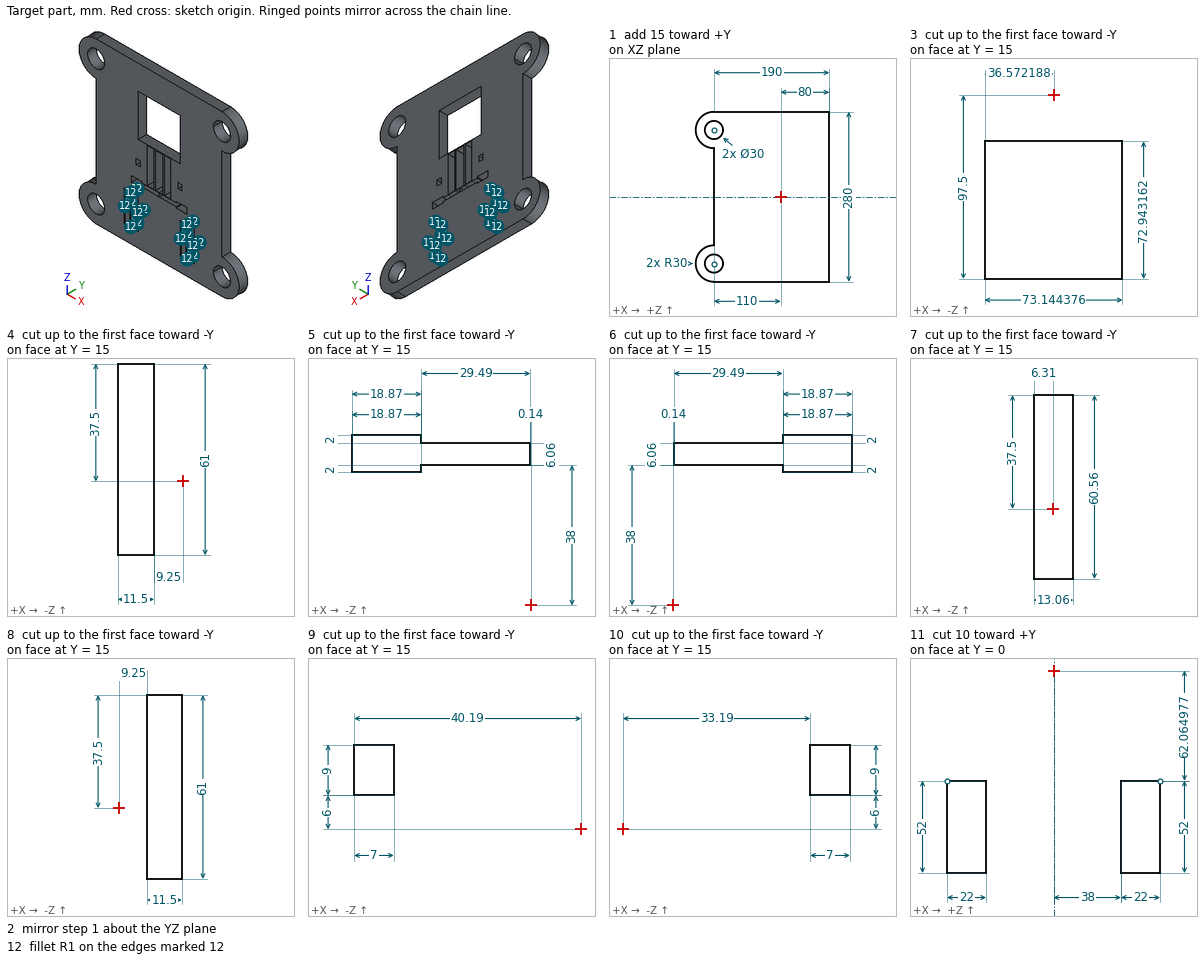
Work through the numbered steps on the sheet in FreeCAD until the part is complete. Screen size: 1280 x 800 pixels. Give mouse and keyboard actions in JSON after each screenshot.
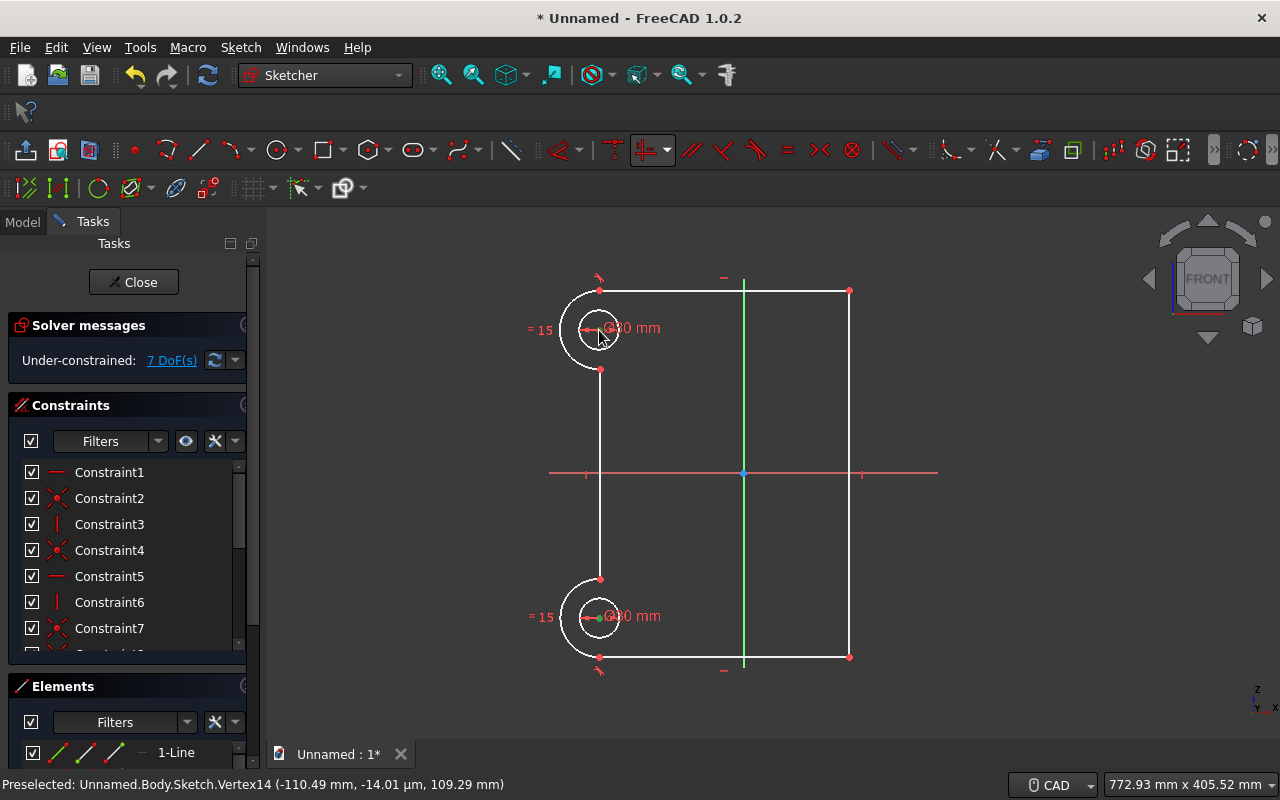
{"action": "left_click", "coordinate": [646, 473]}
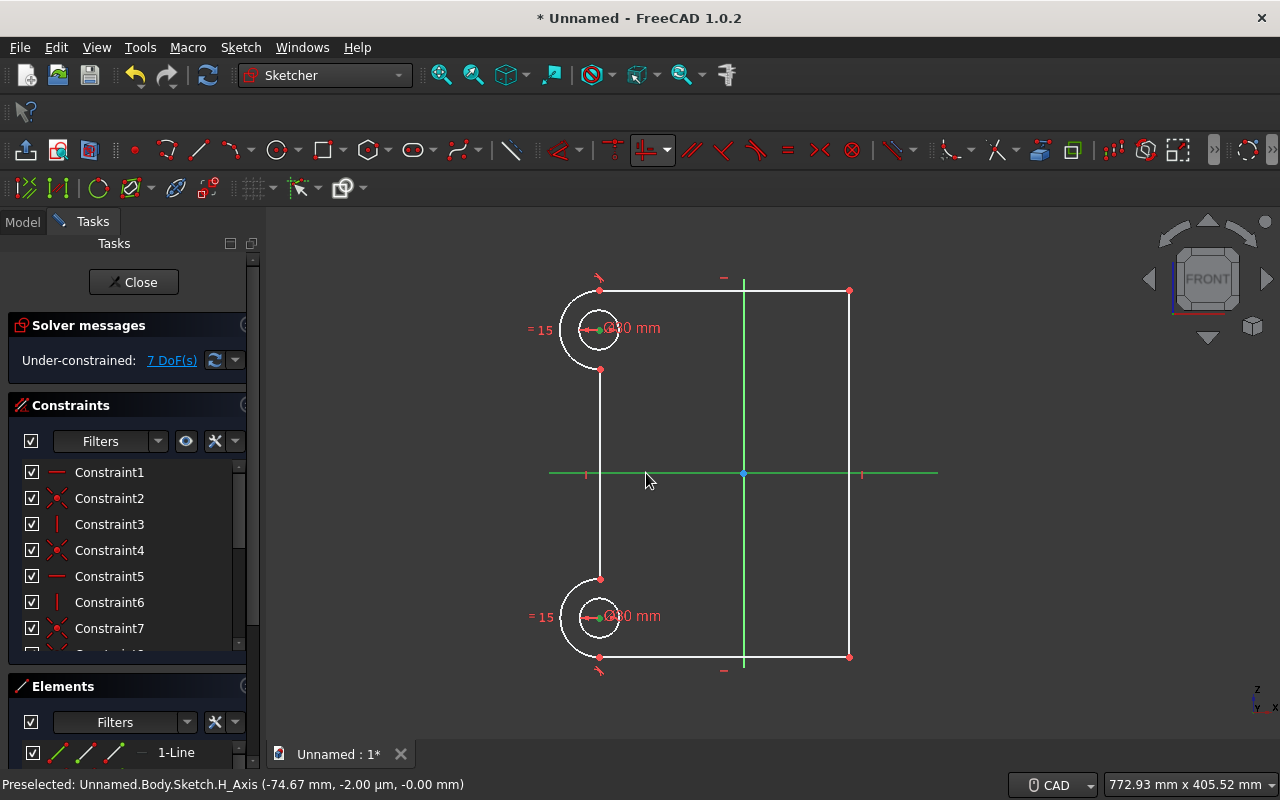
{"action": "left_click", "coordinate": [820, 150]}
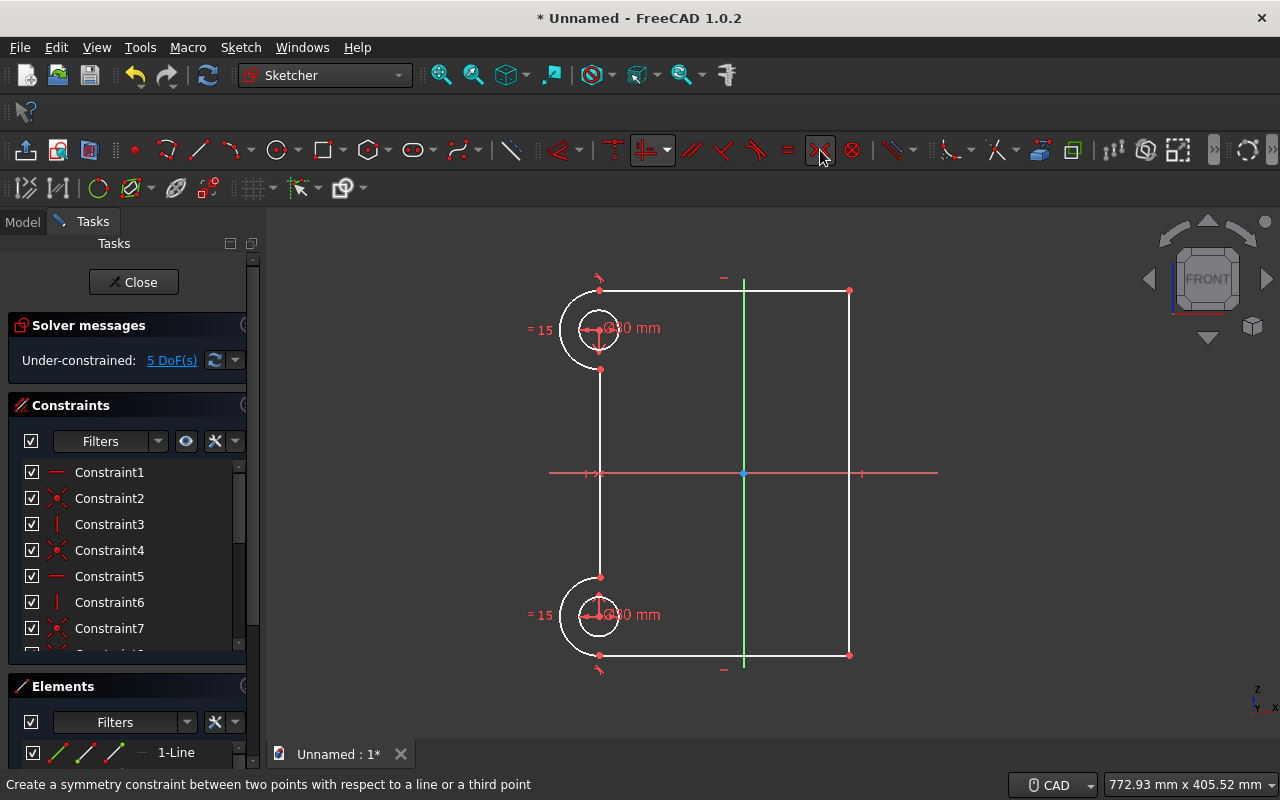
{"action": "left_click", "coordinate": [558, 150]}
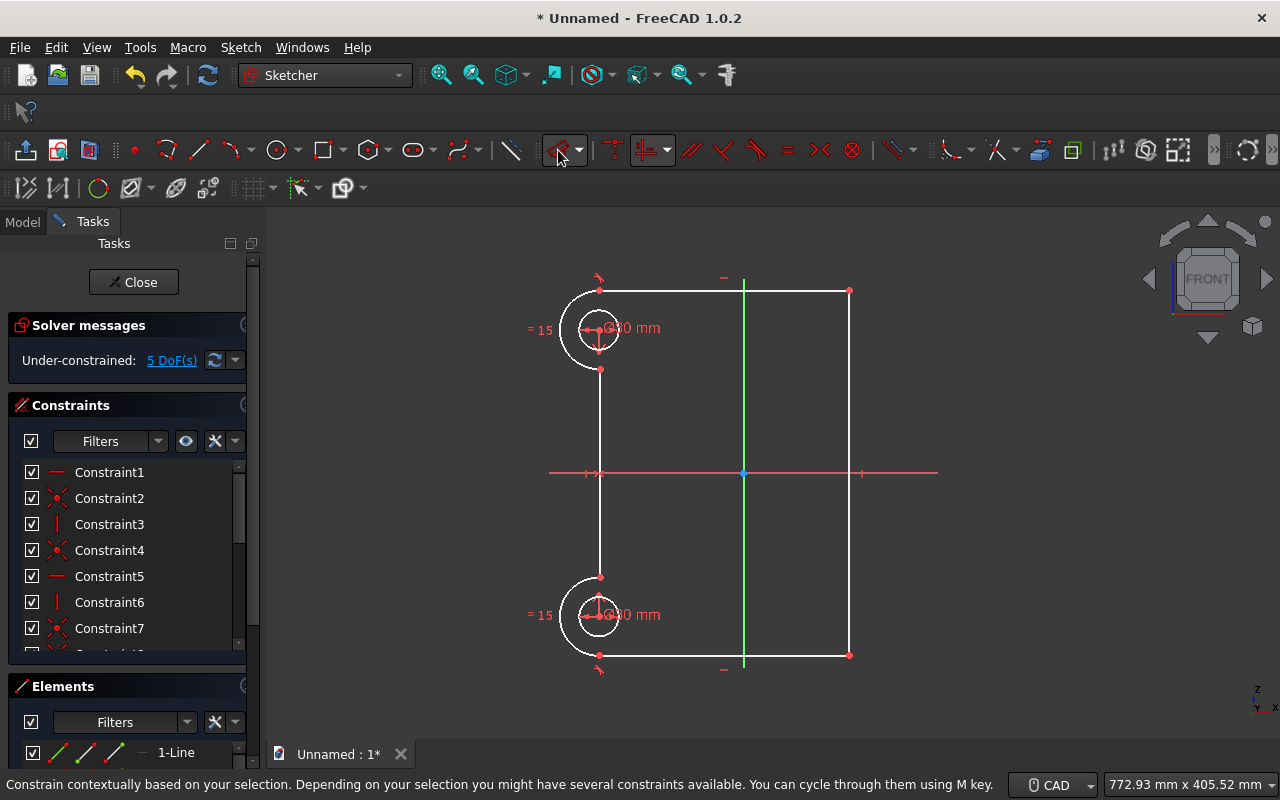
{"action": "left_click", "coordinate": [568, 593]}
{"action": "left_click", "coordinate": [543, 574]}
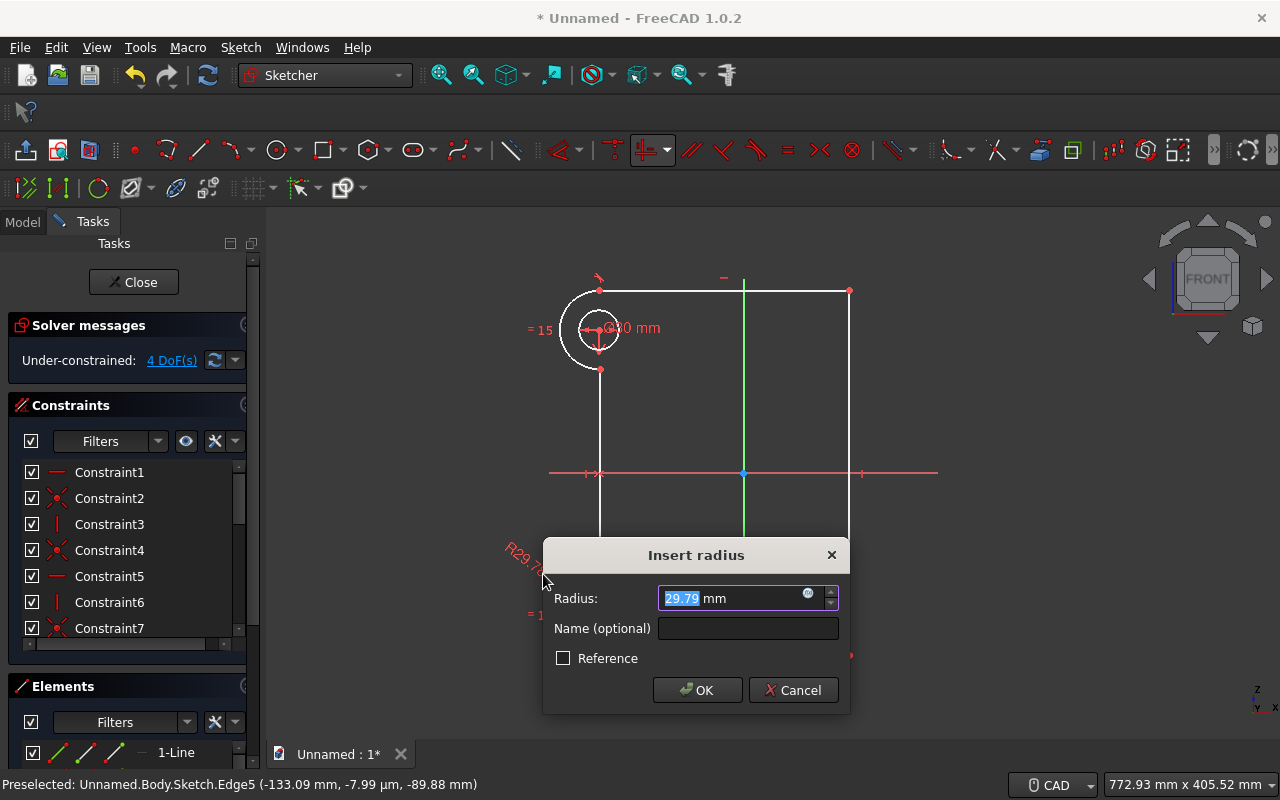
{"action": "type", "text": "30"}
{"action": "key", "text": "Return"}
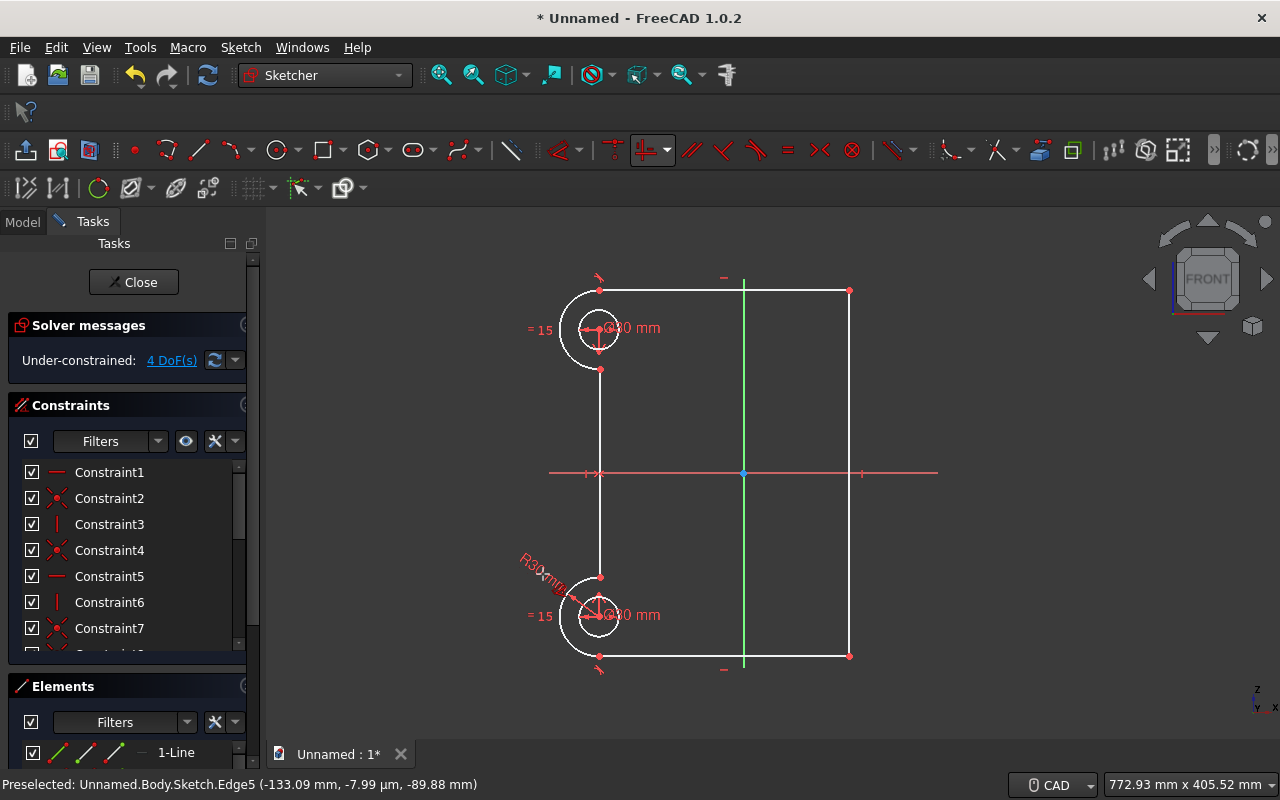
{"action": "left_click", "coordinate": [674, 290]}
{"action": "left_click", "coordinate": [724, 256]}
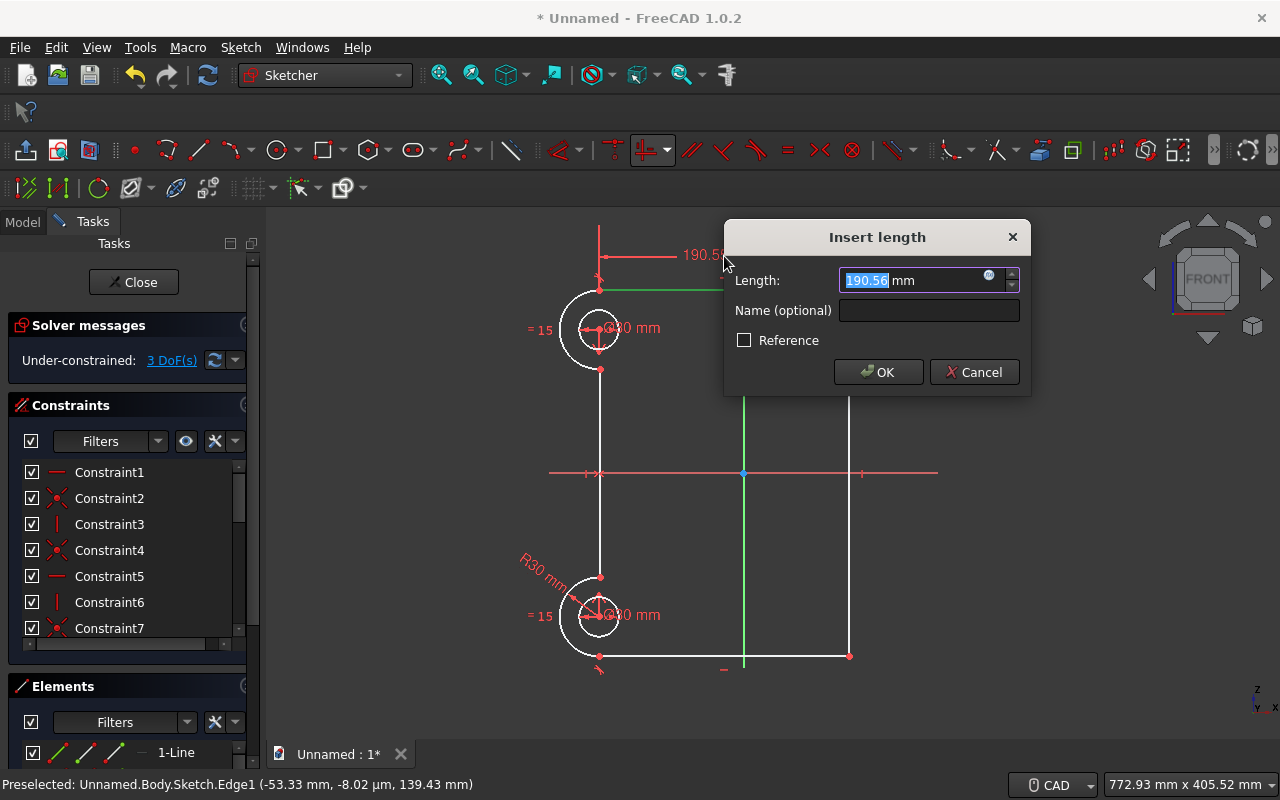
{"action": "type", "text": "190"}
{"action": "key", "text": "Return"}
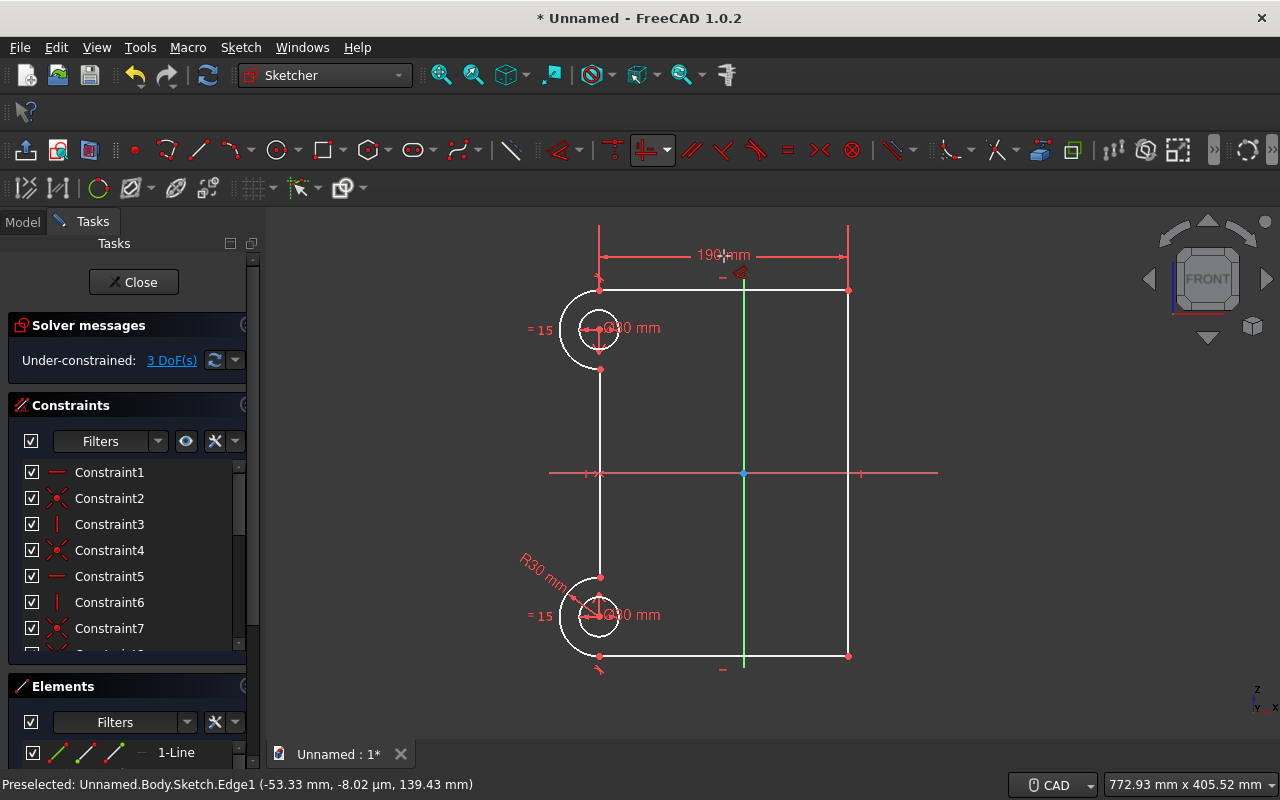
{"action": "left_click", "coordinate": [848, 400]}
{"action": "left_click", "coordinate": [882, 389]}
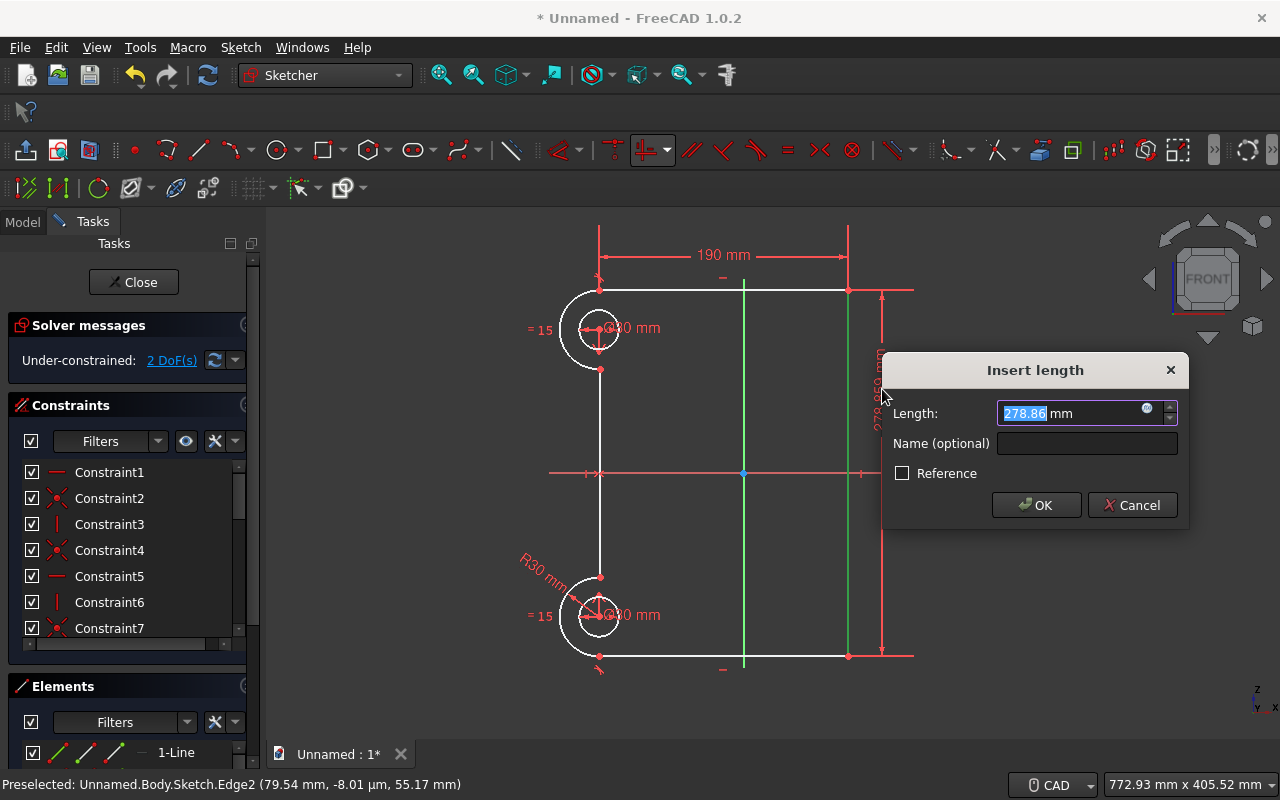
{"action": "type", "text": "280"}
{"action": "key", "text": "Return"}